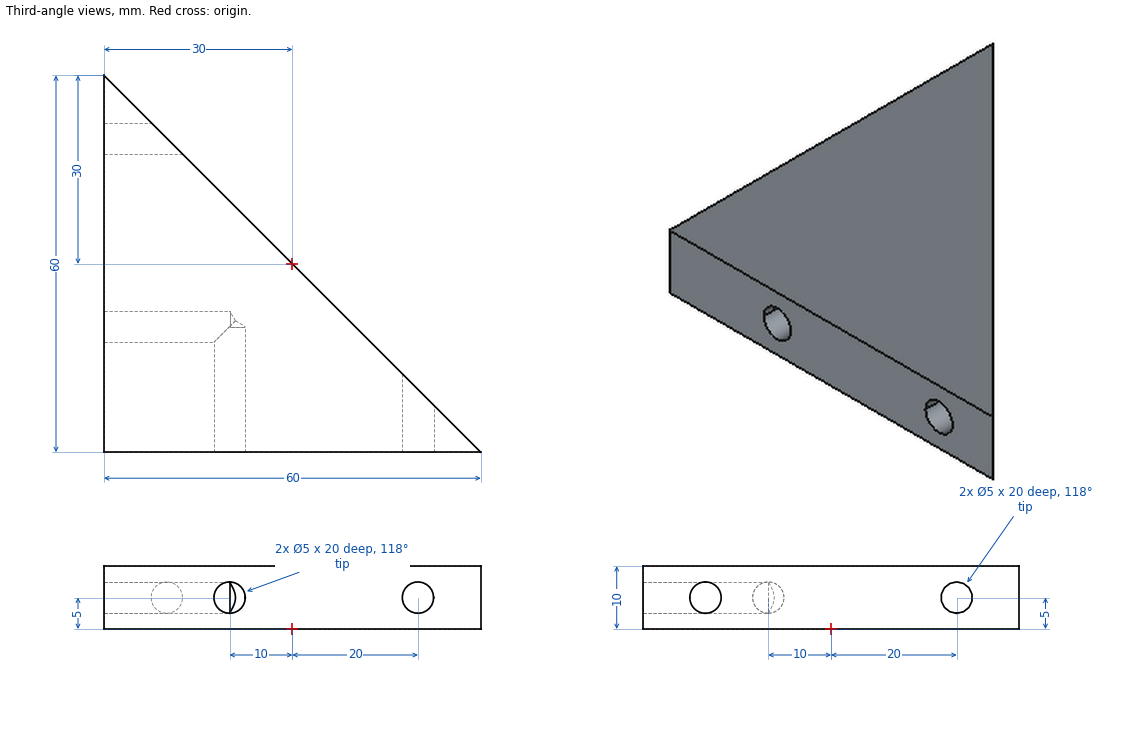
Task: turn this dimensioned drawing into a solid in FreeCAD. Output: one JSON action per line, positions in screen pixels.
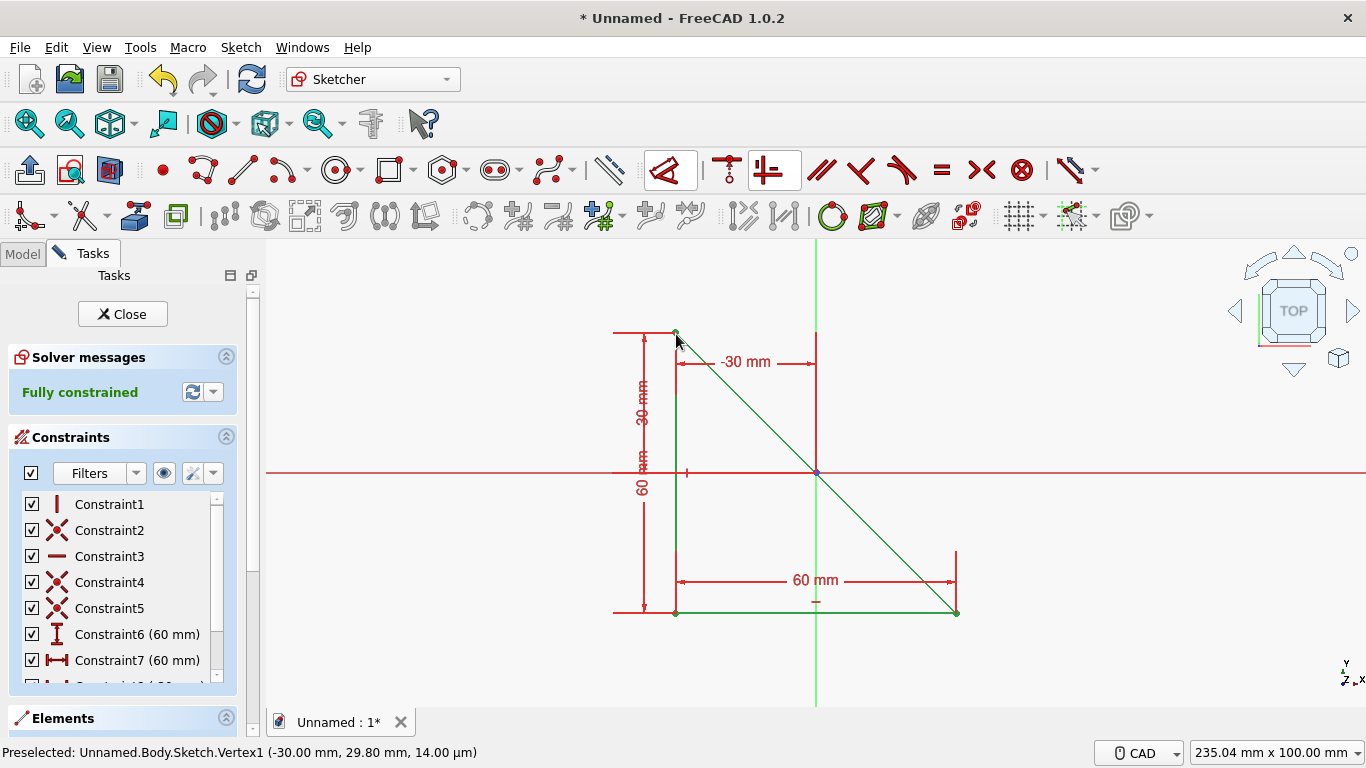
{"action": "left_click", "coordinate": [123, 314]}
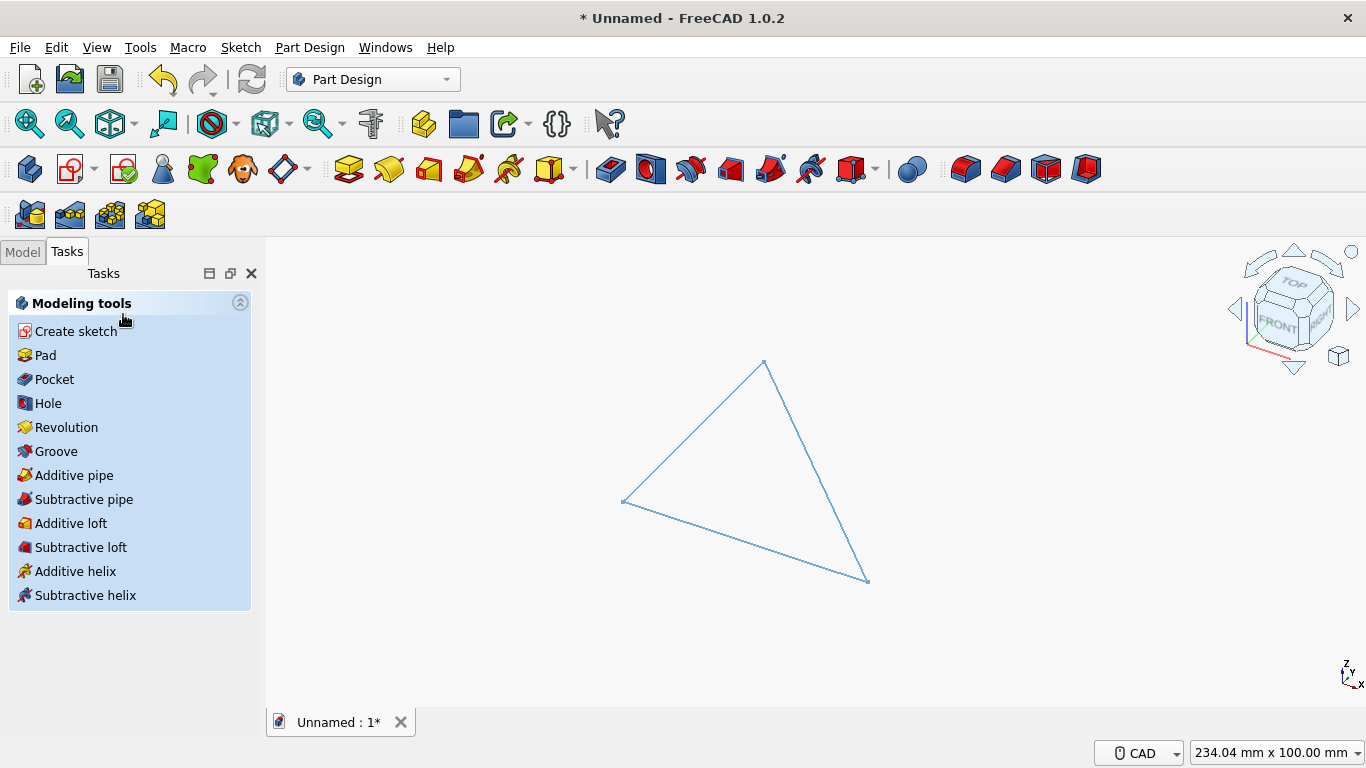
{"action": "left_click", "coordinate": [350, 170]}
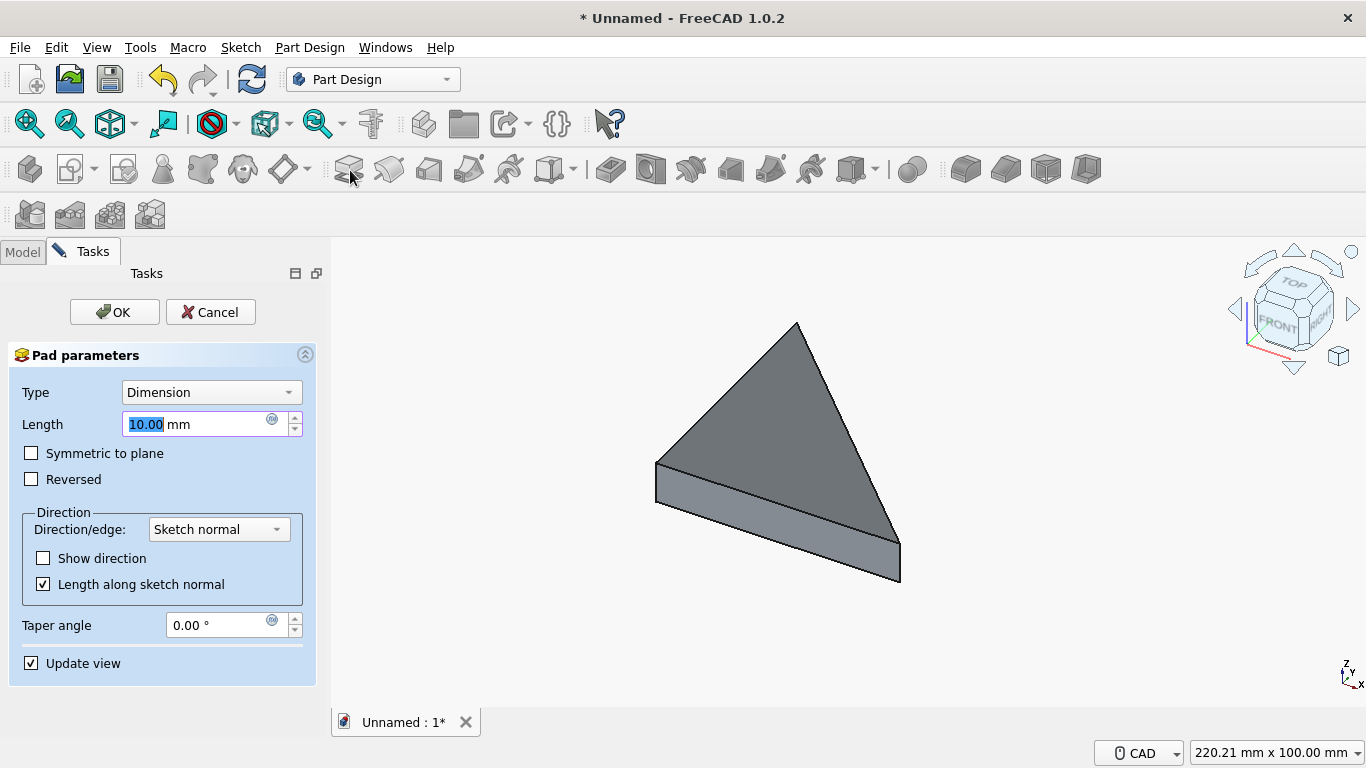
{"action": "type", "text": "10"}
{"action": "key", "text": "Tab"}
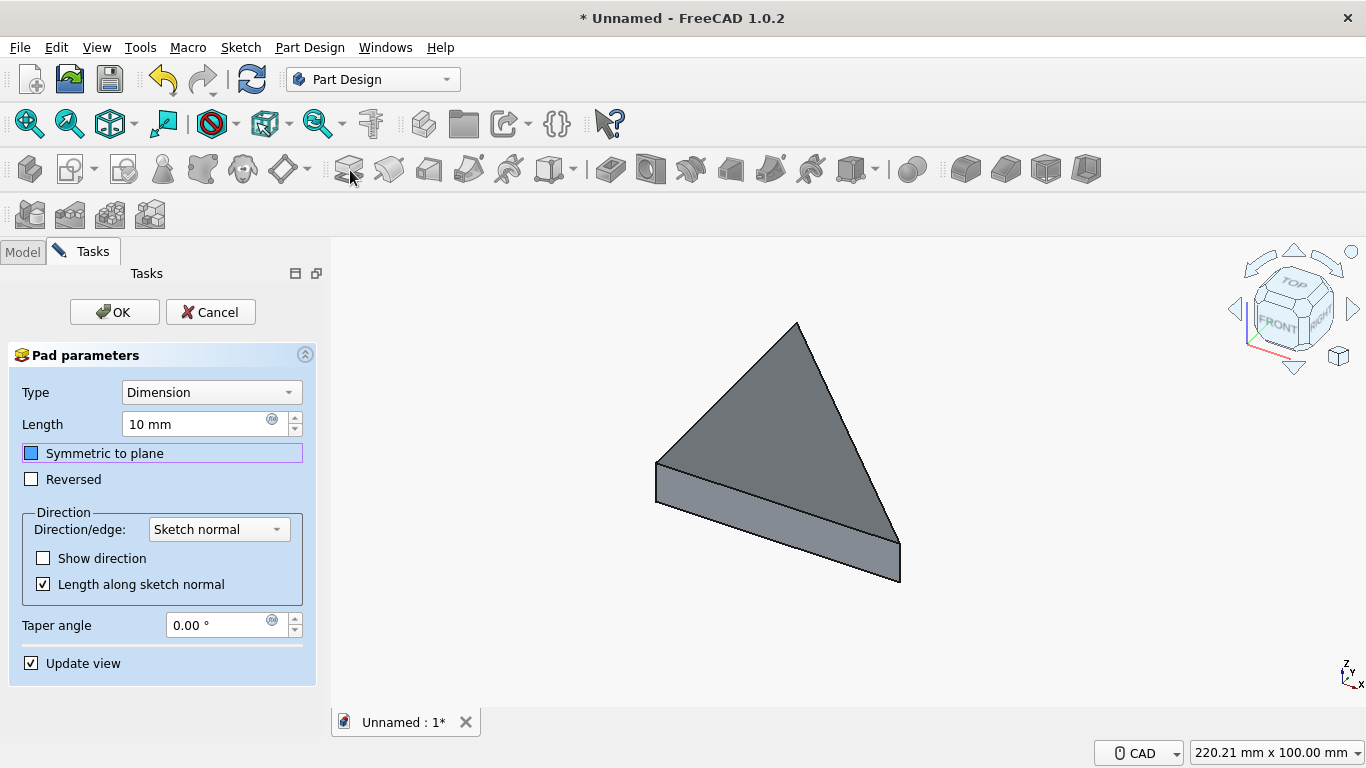
{"action": "left_click", "coordinate": [115, 312]}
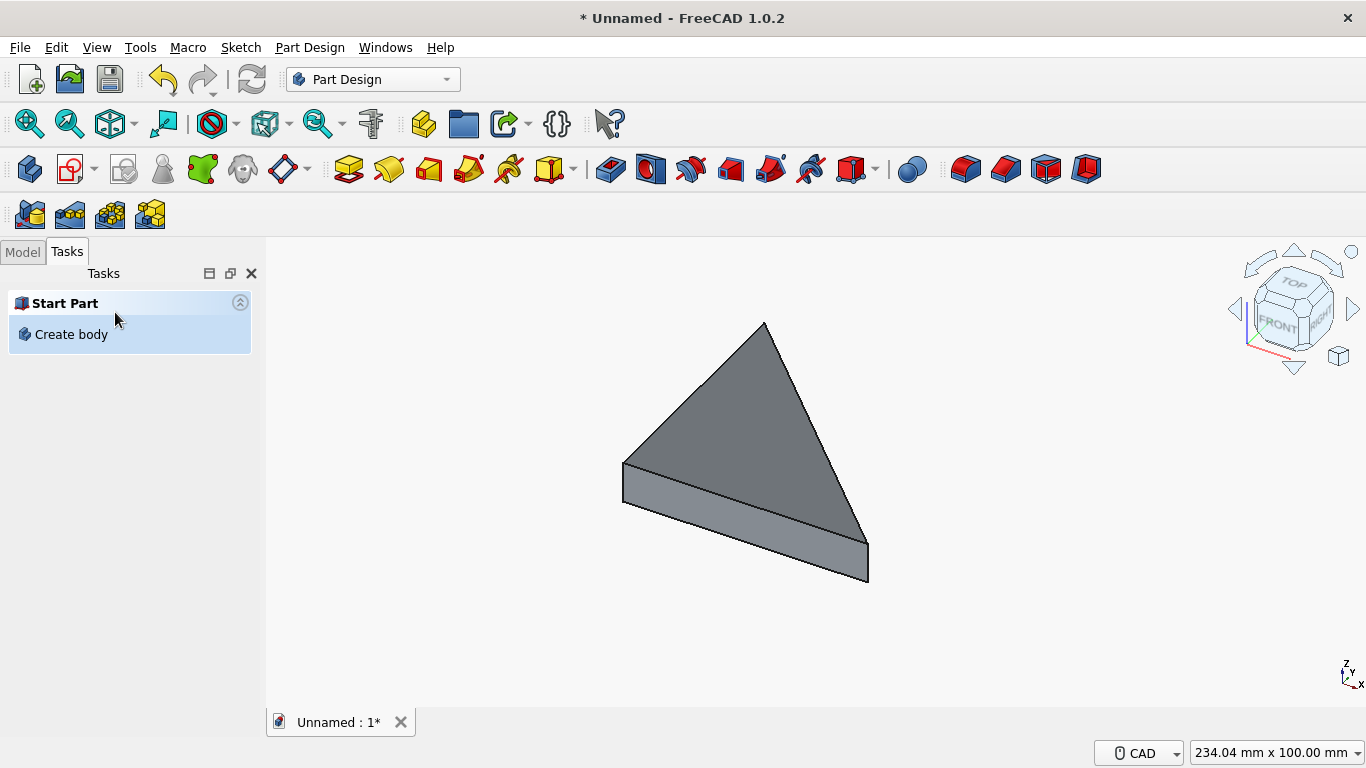
{"action": "left_click", "coordinate": [815, 545]}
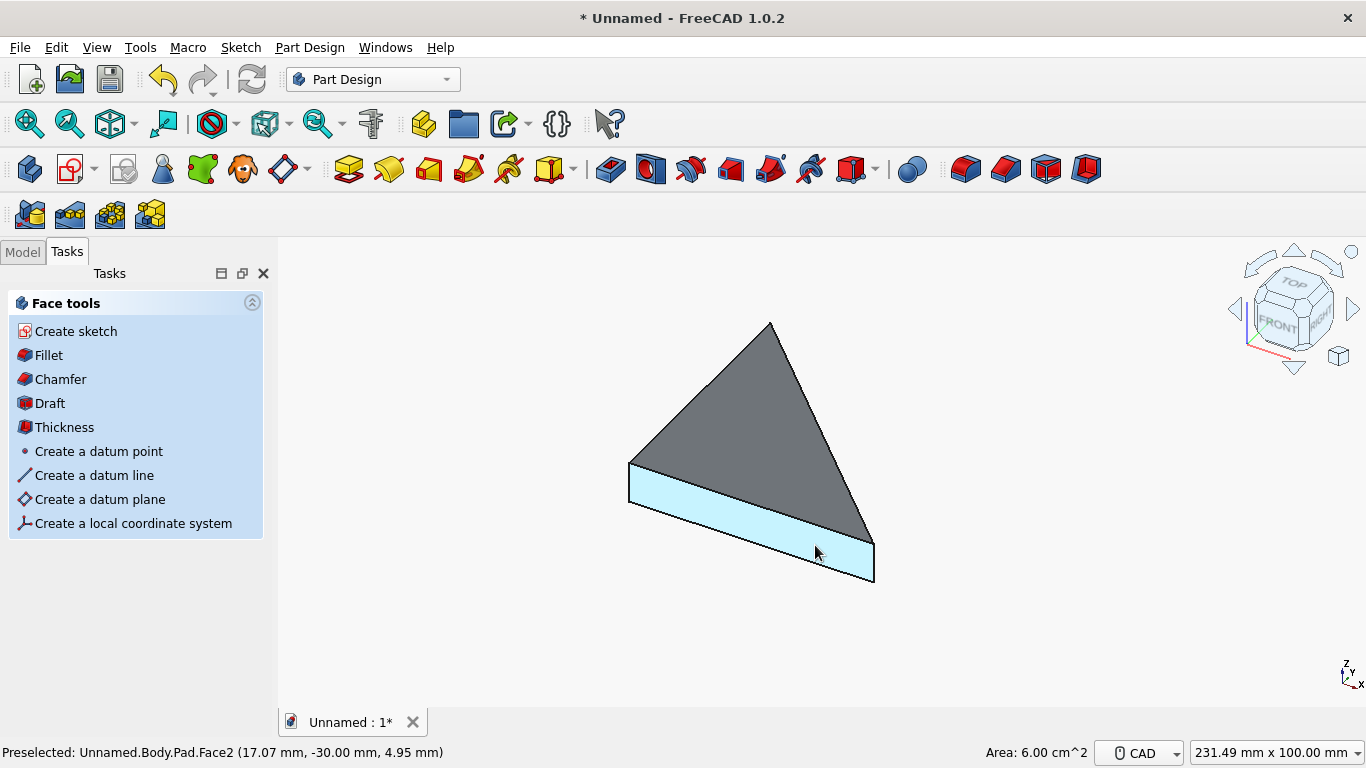
{"action": "left_click", "coordinate": [70, 170]}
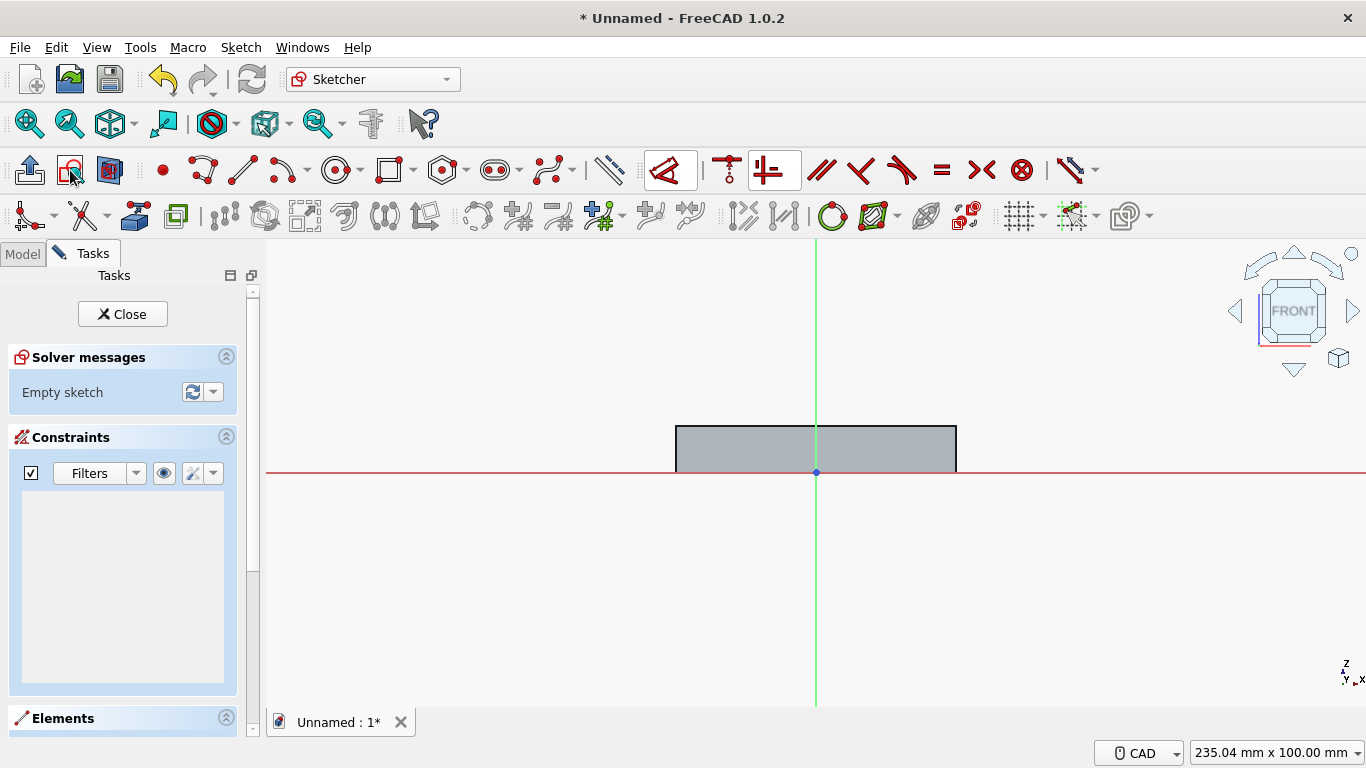
{"action": "scroll", "coordinate": [869, 450], "scroll_direction": "up", "scroll_amount": 7}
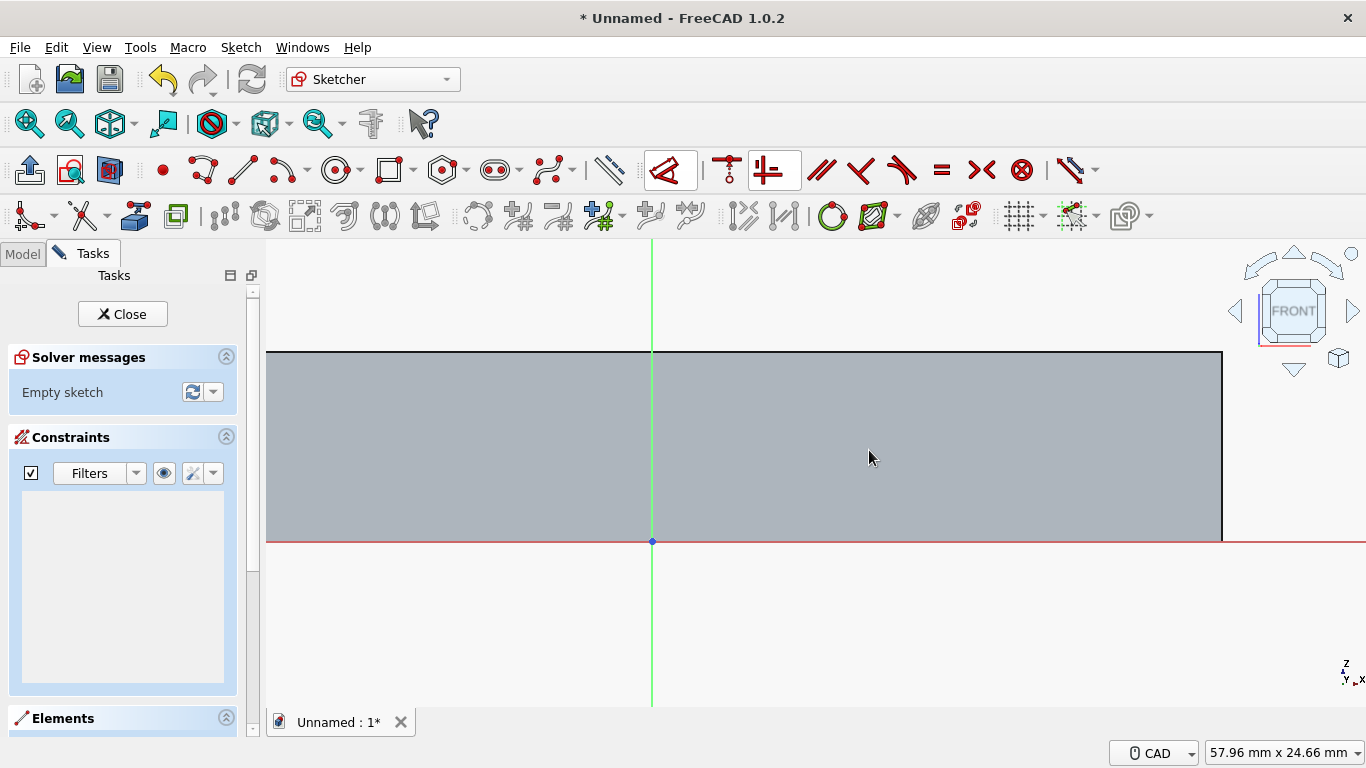
{"action": "left_click", "coordinate": [336, 170]}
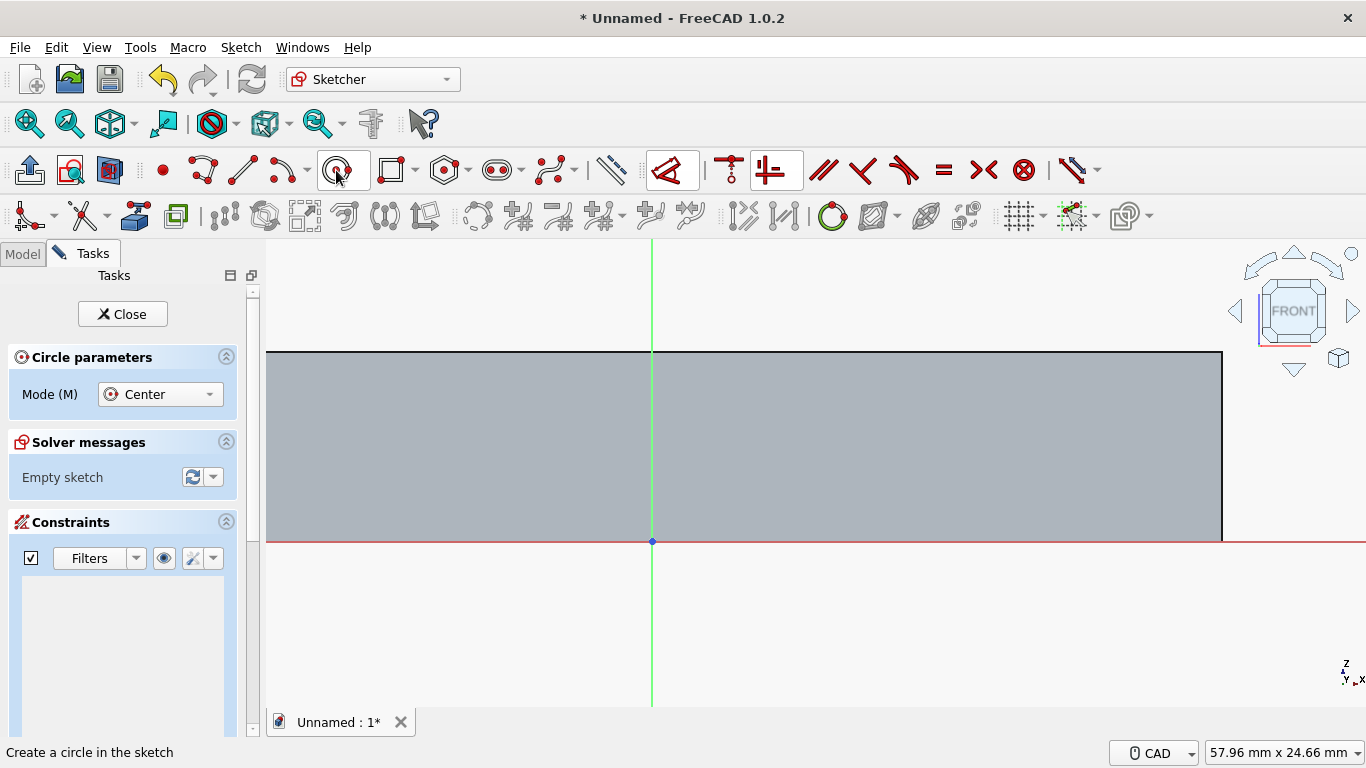
{"action": "left_click", "coordinate": [463, 447]}
{"action": "mouse_move", "coordinate": [496, 413]}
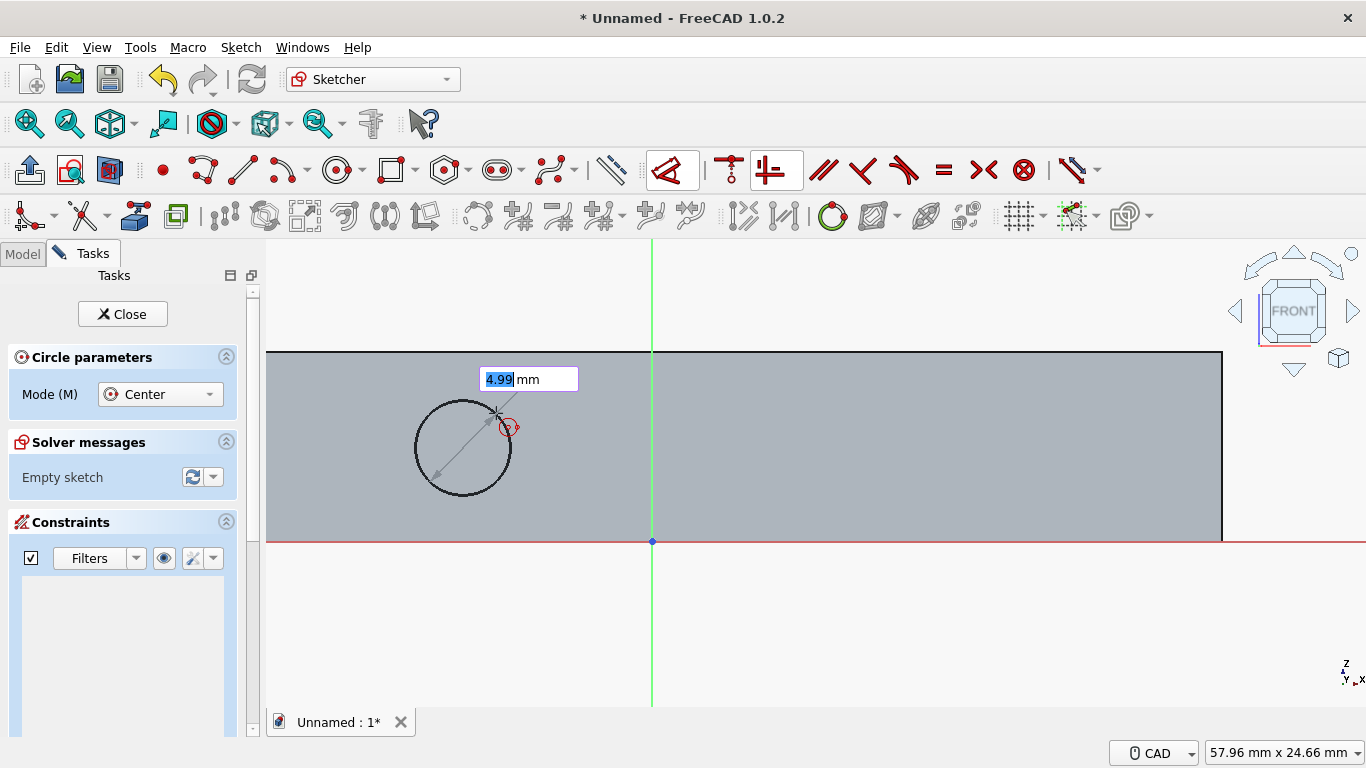
{"action": "type", "text": "5"}
{"action": "key", "text": "Return"}